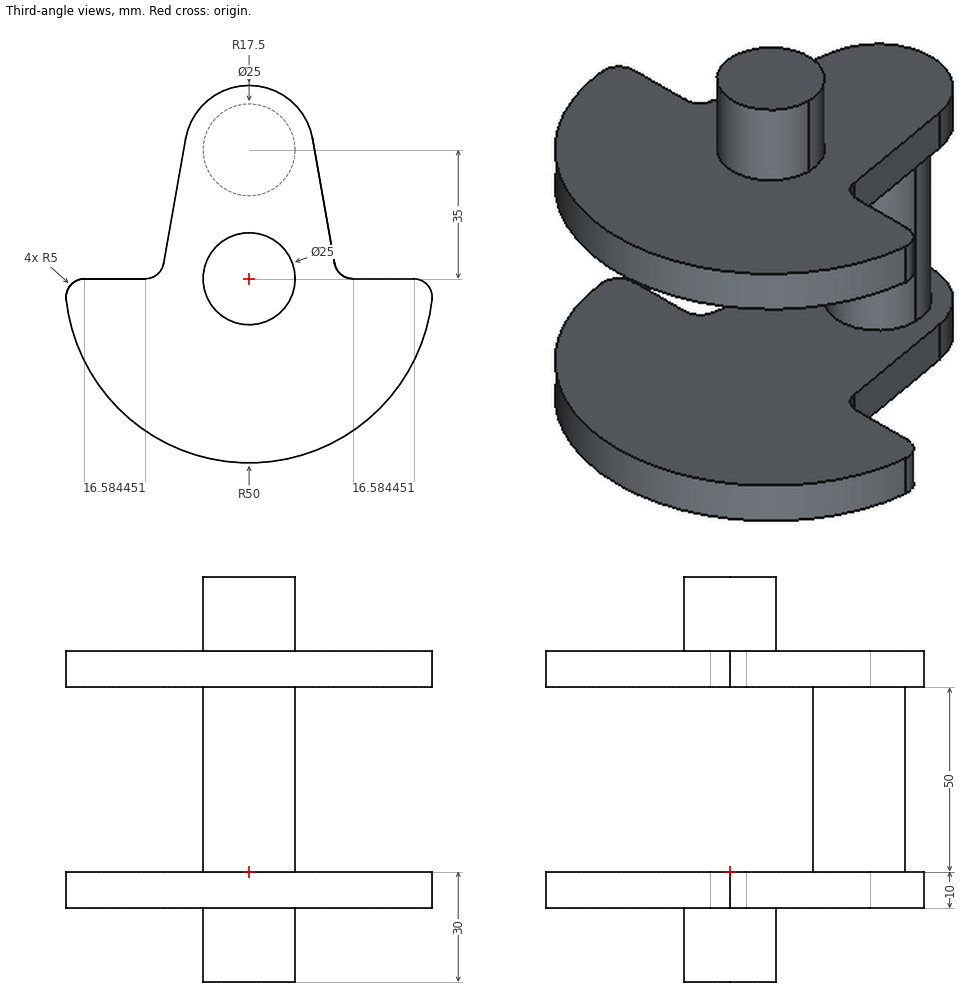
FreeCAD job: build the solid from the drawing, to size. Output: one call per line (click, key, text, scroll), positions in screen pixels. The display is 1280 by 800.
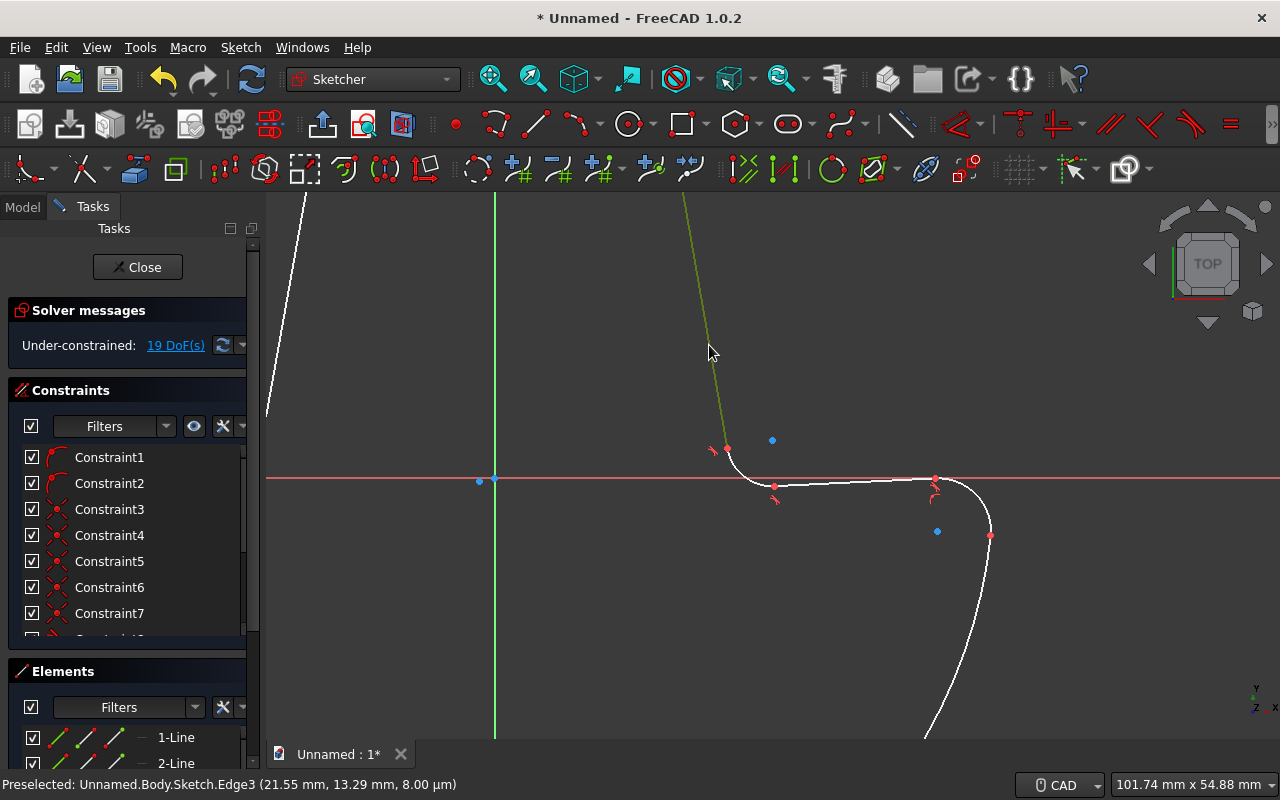
scroll(827, 465, down, 5)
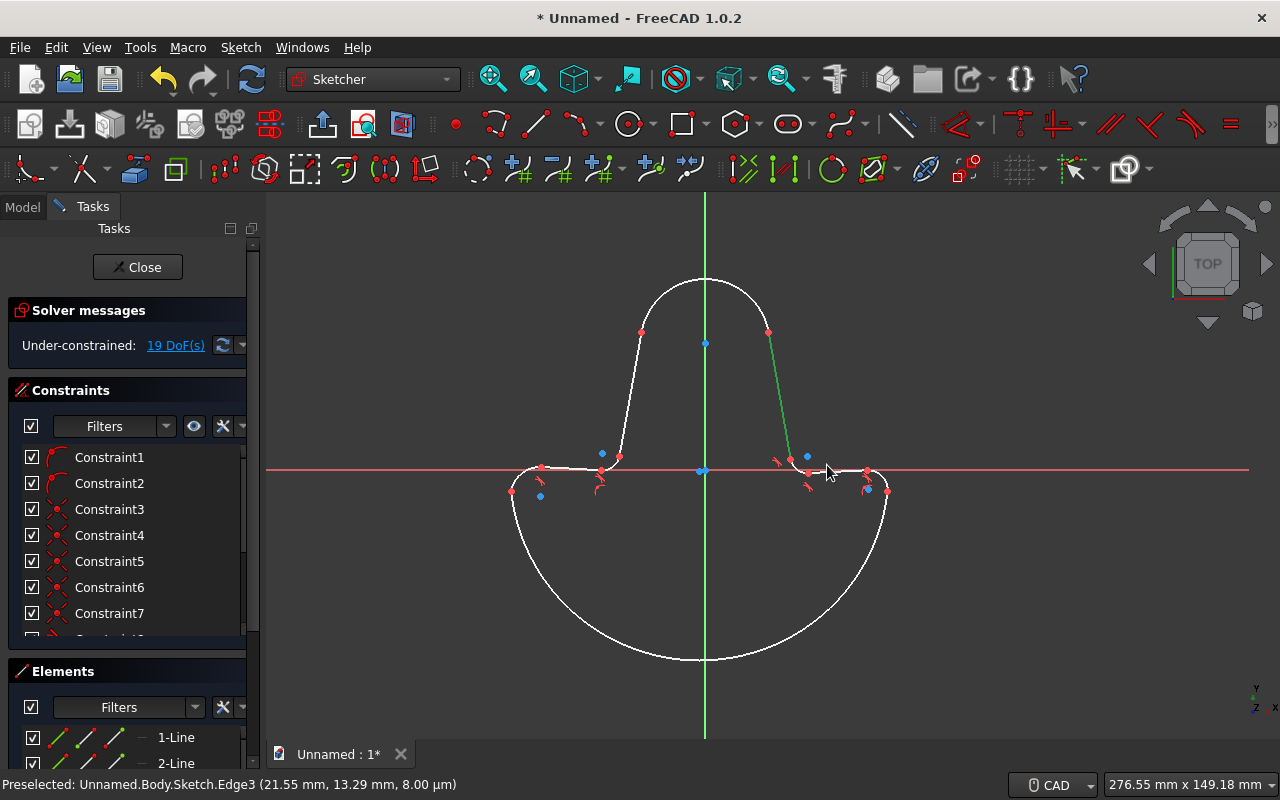
click(739, 289)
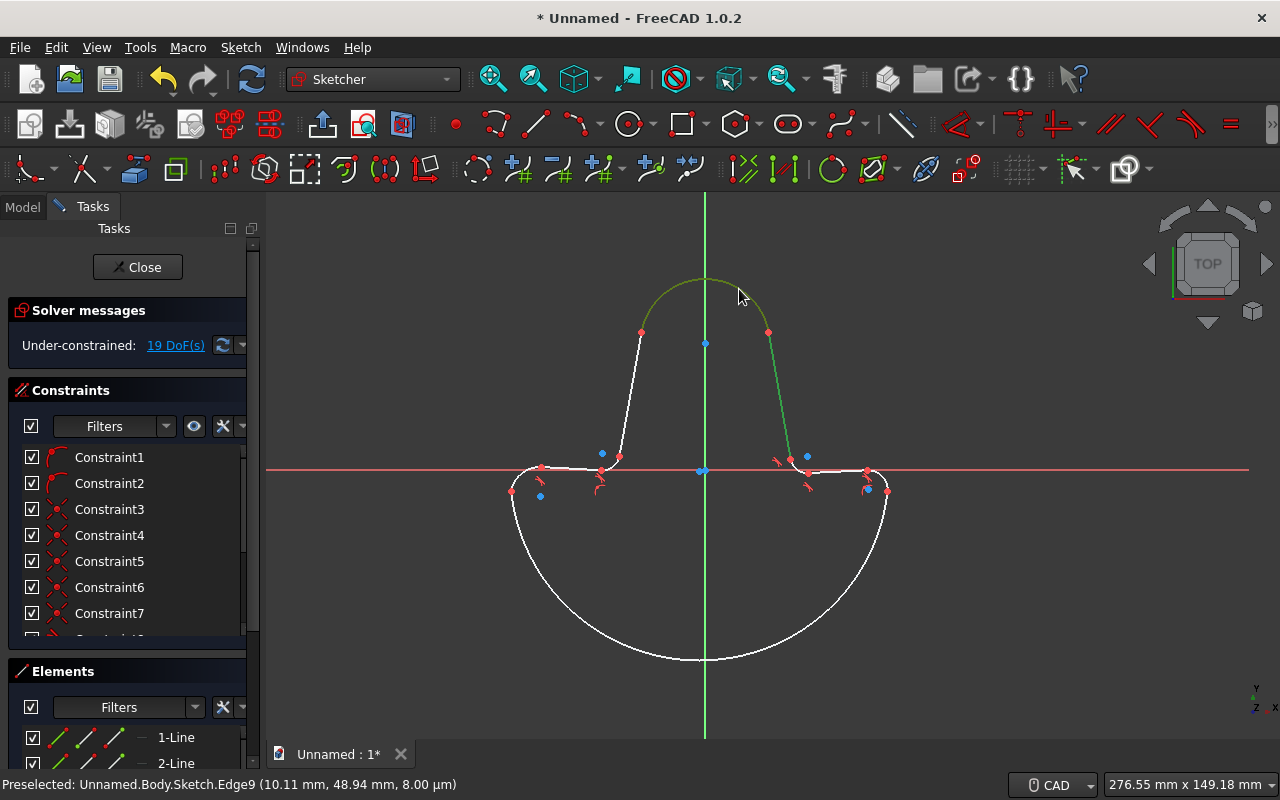
key(t)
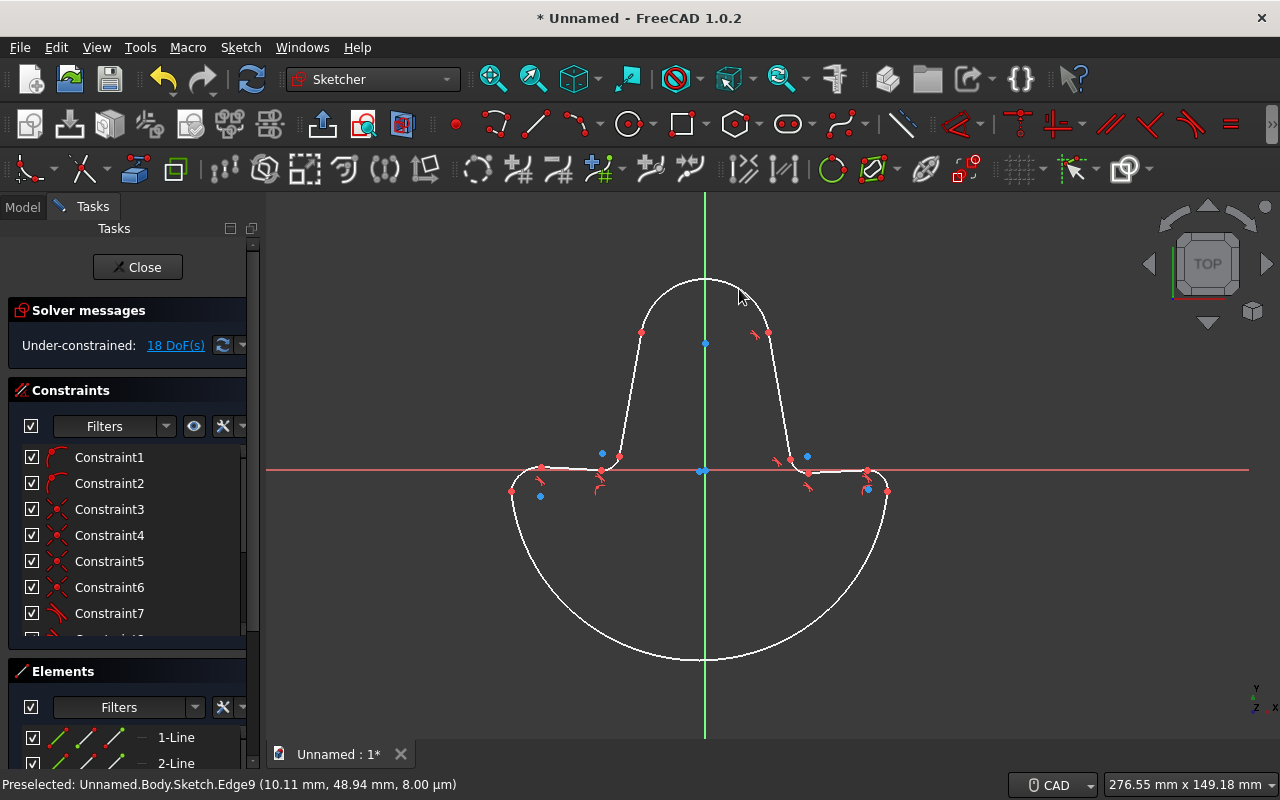
click(635, 369)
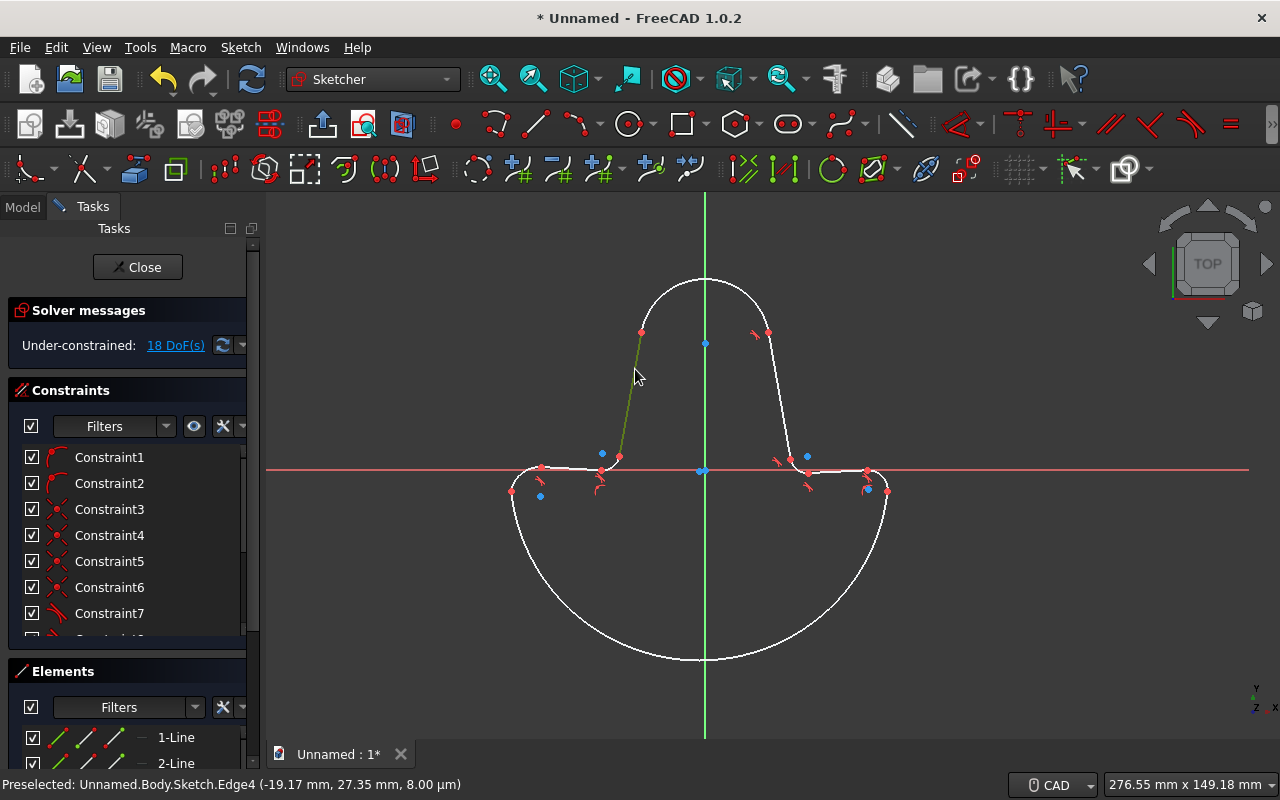
click(739, 289)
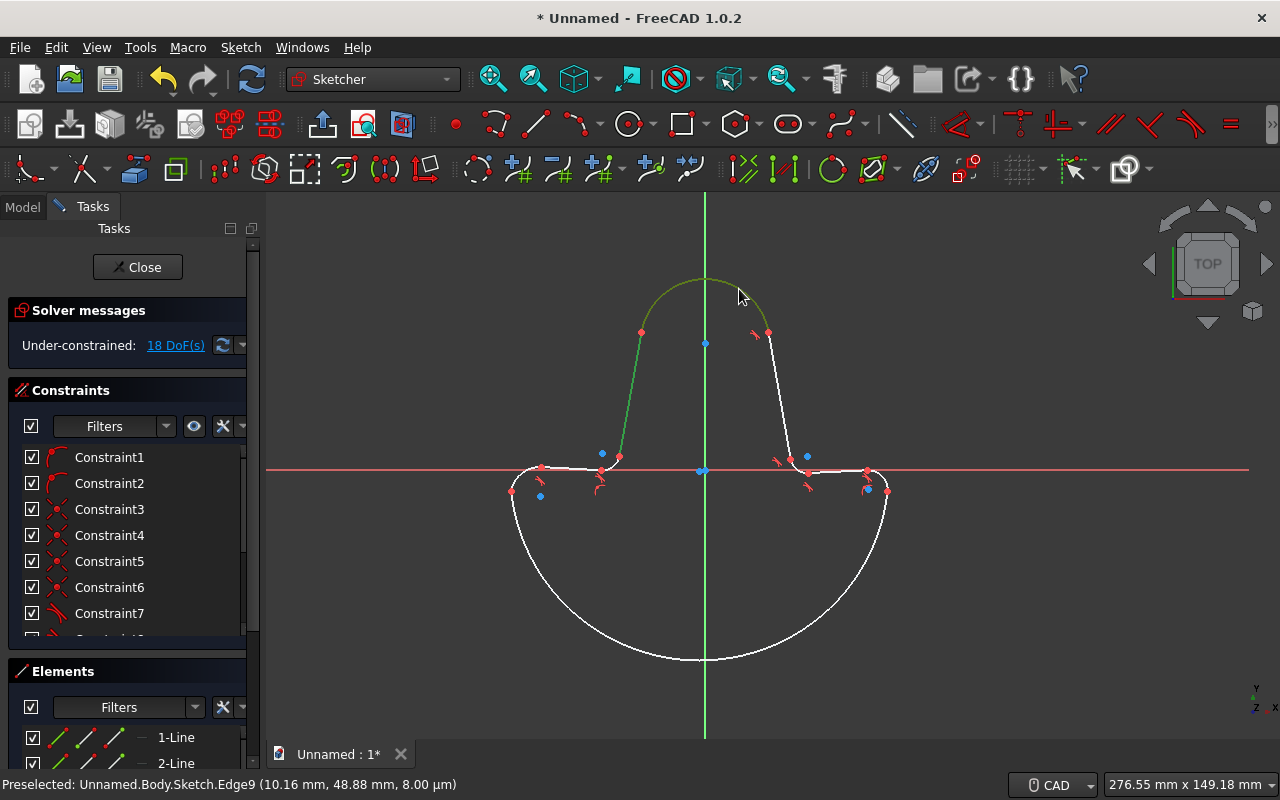
key(t)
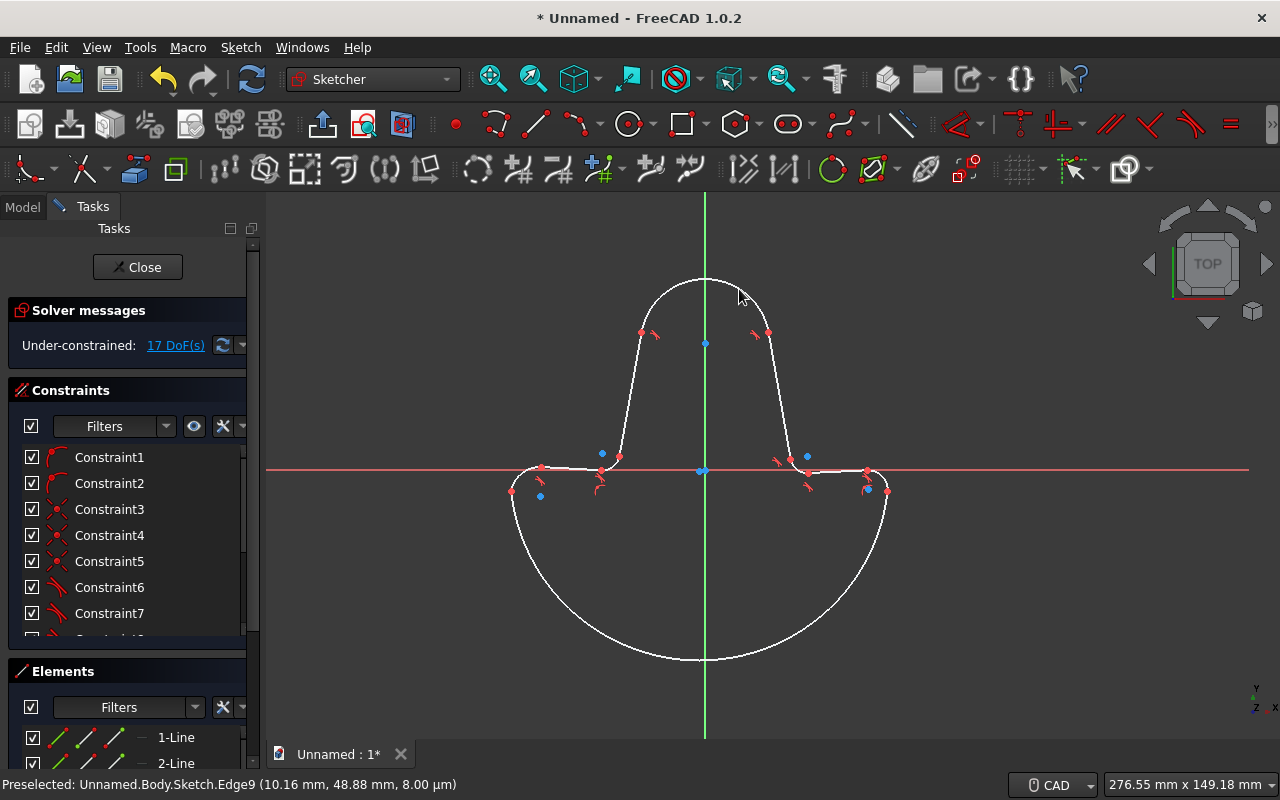
click(635, 369)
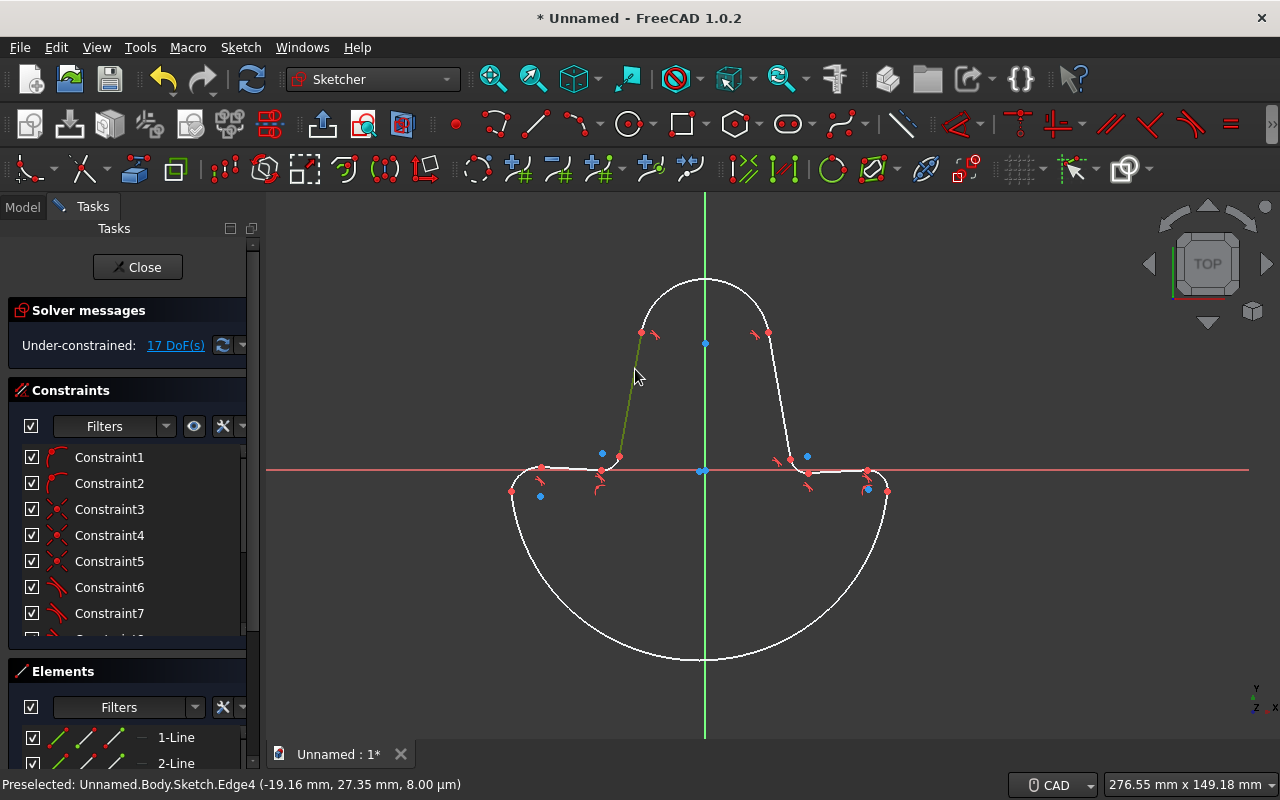
click(613, 467)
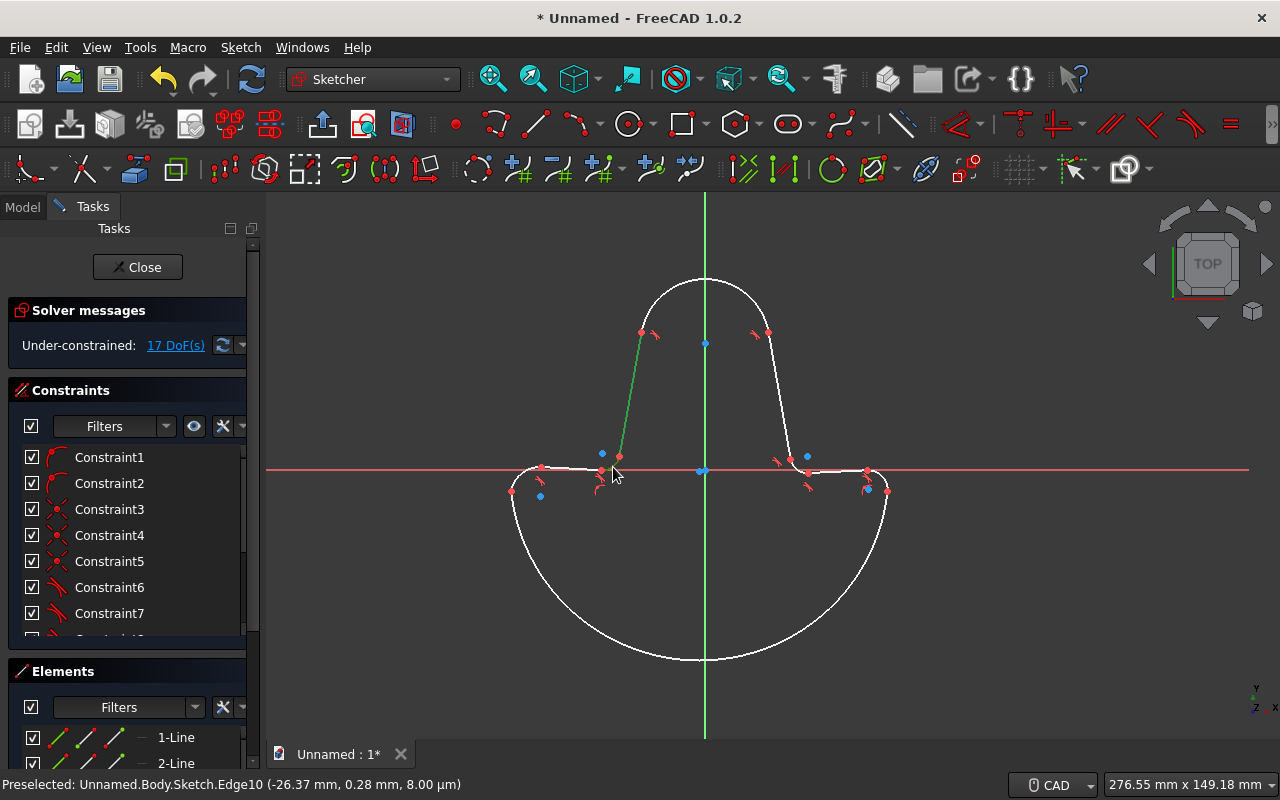
key(t)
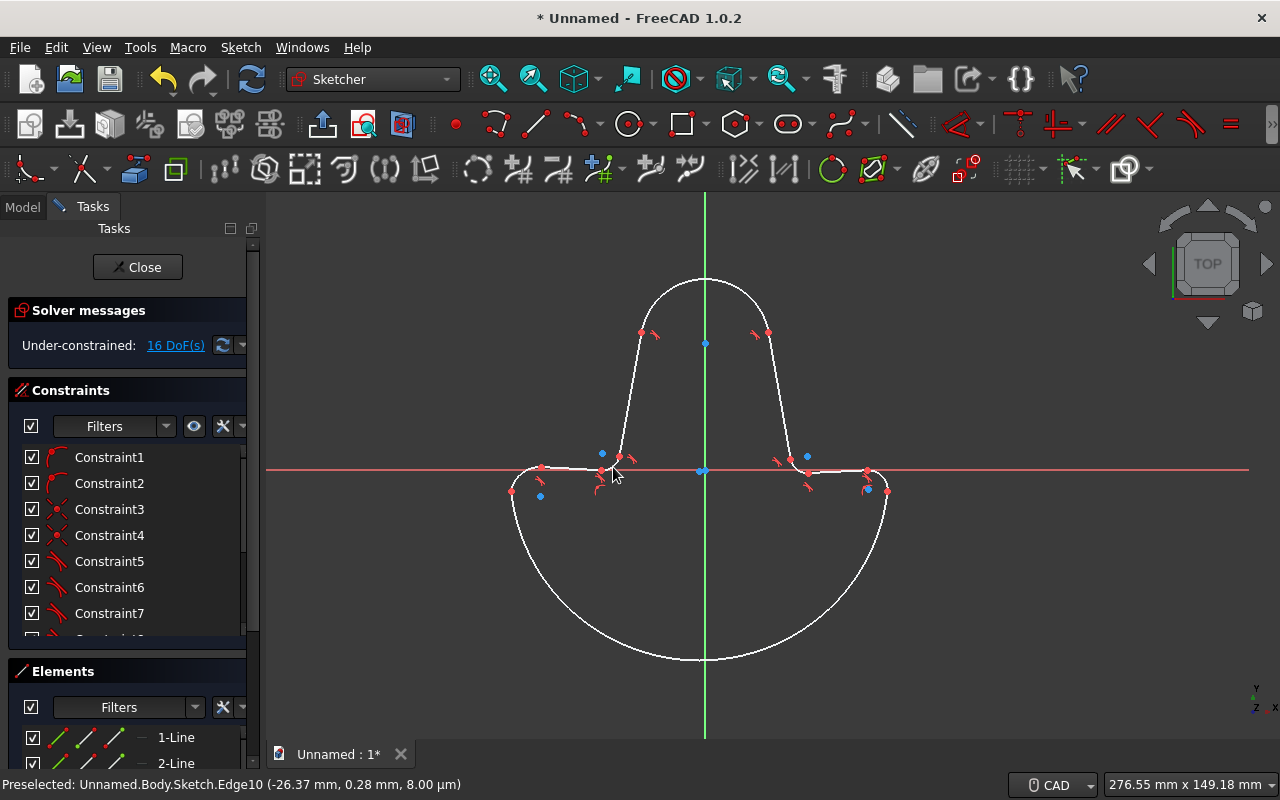
click(529, 469)